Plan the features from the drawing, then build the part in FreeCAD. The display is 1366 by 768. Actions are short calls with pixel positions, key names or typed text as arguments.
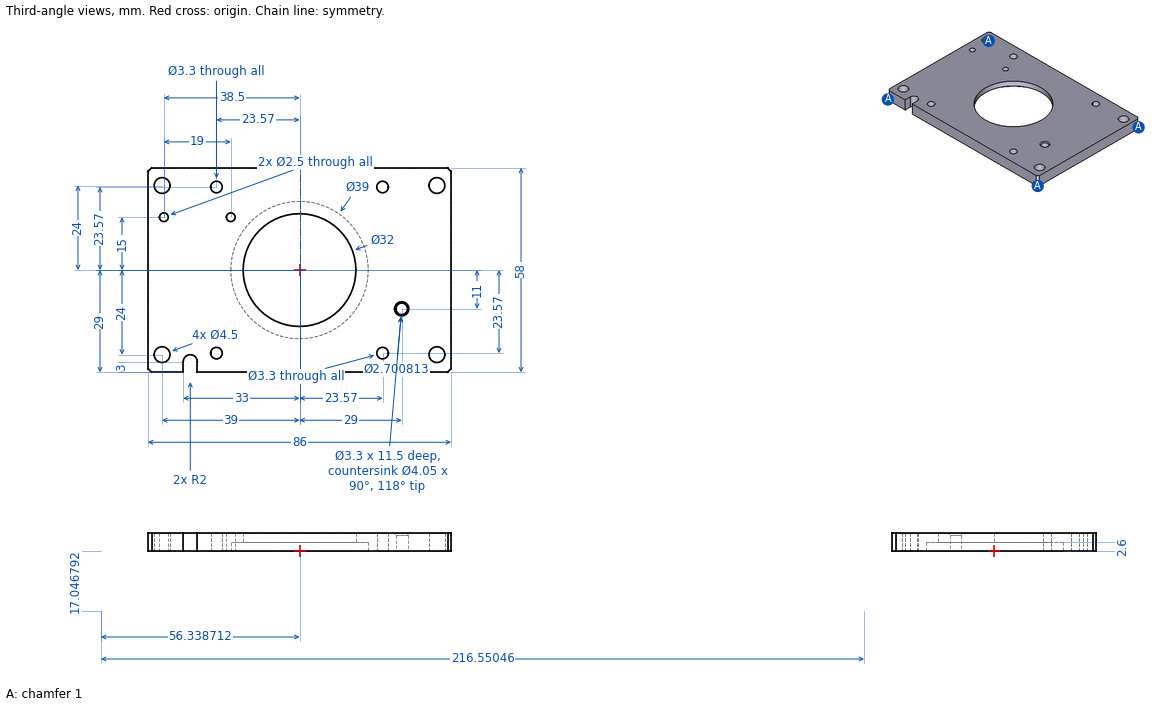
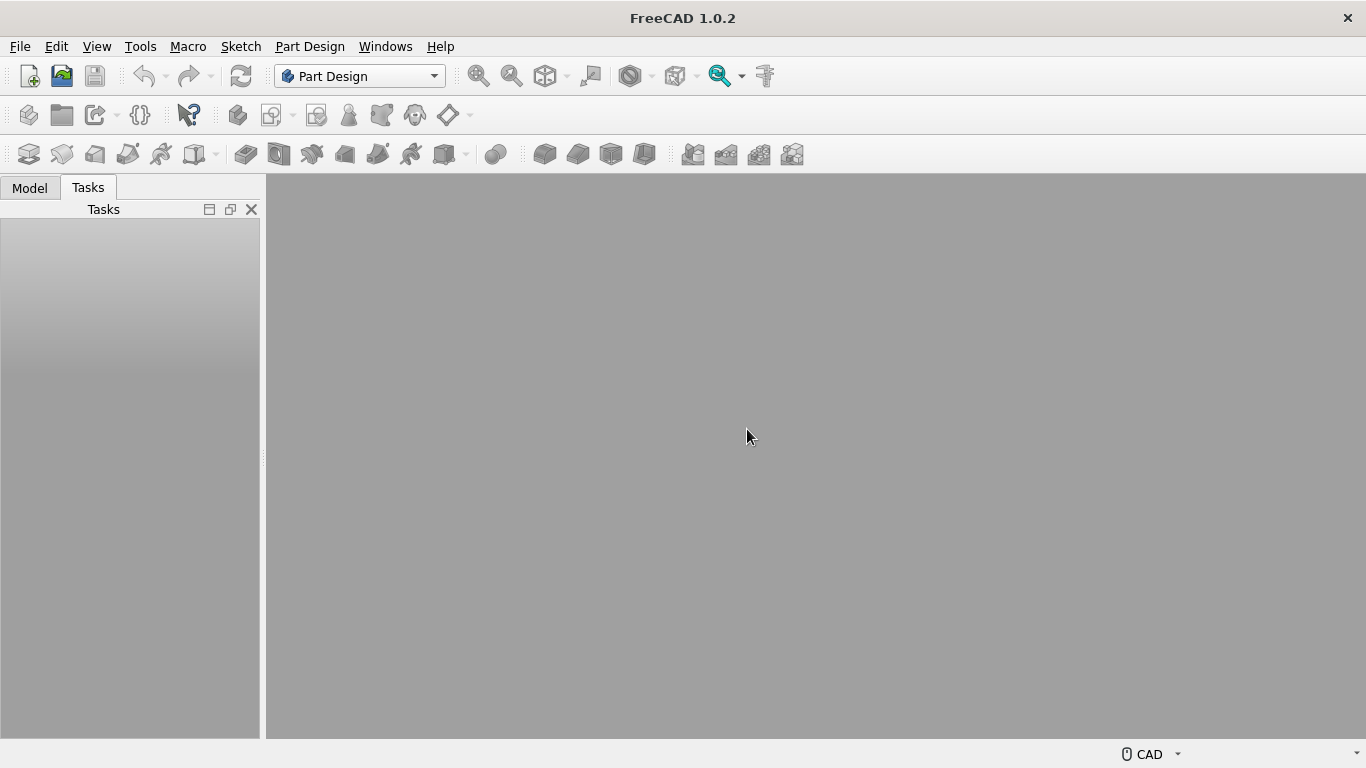
click(29, 76)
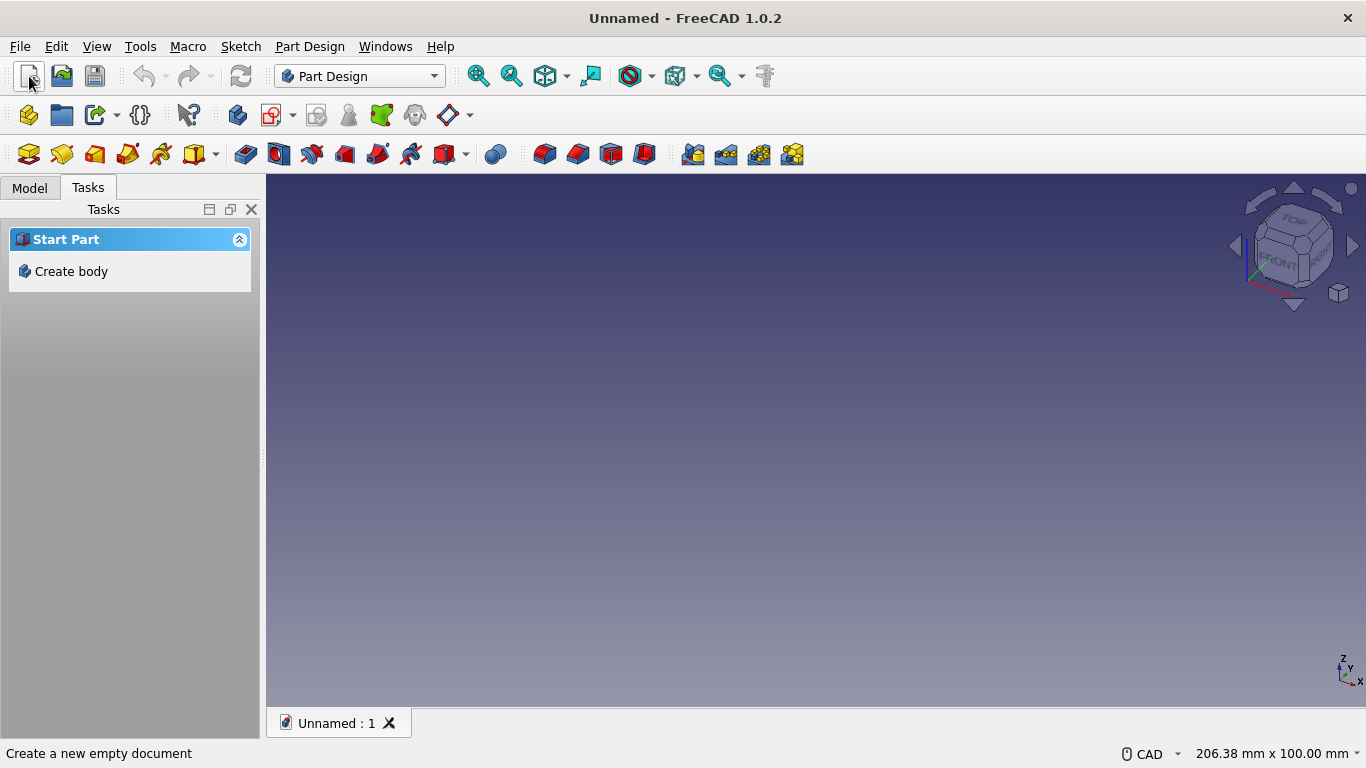
click(270, 116)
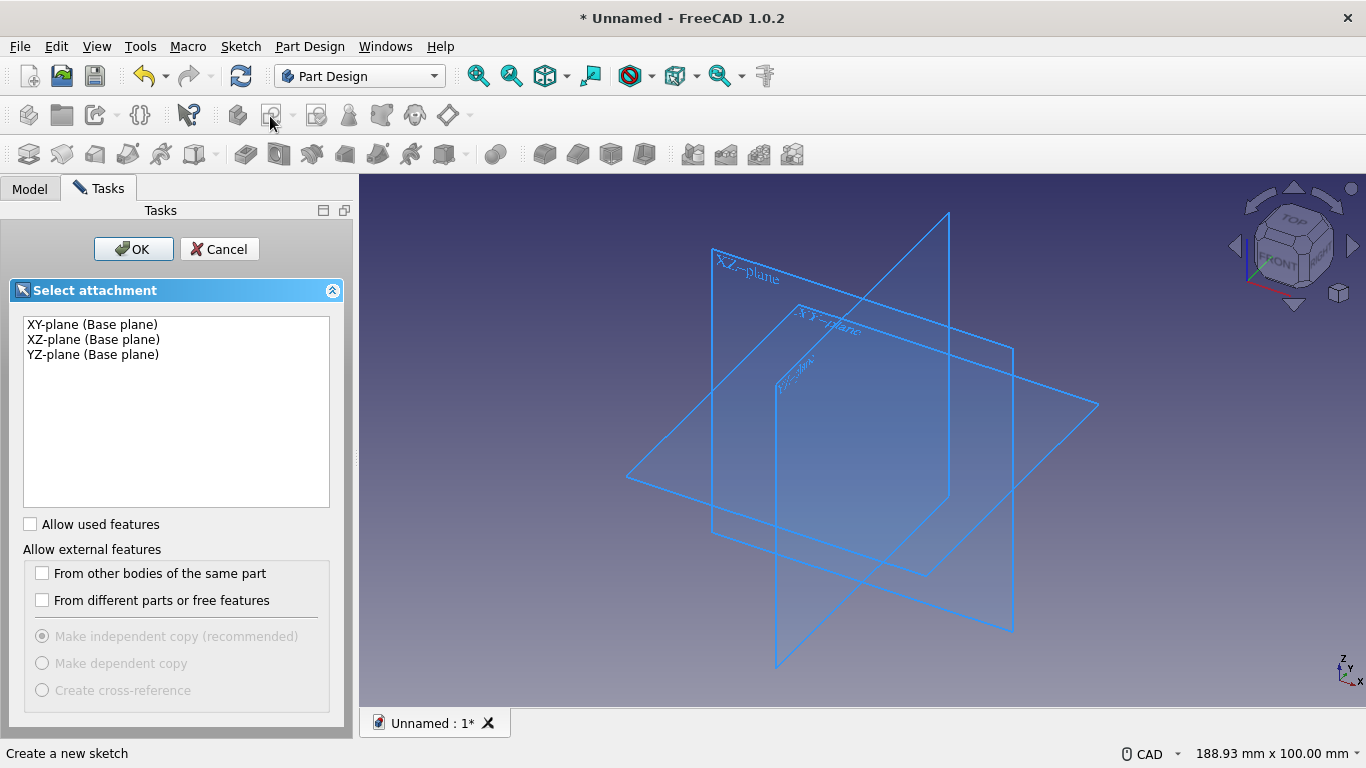
click(84, 324)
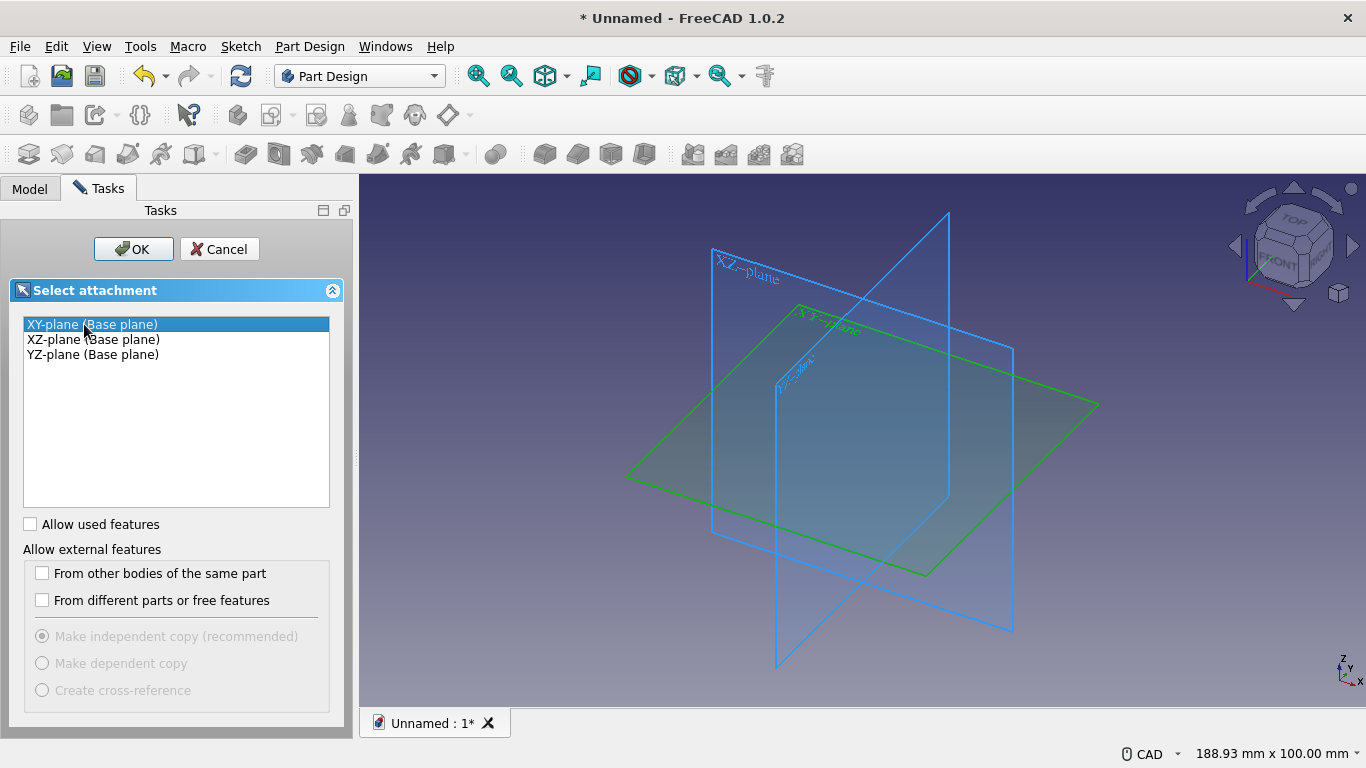
click(134, 249)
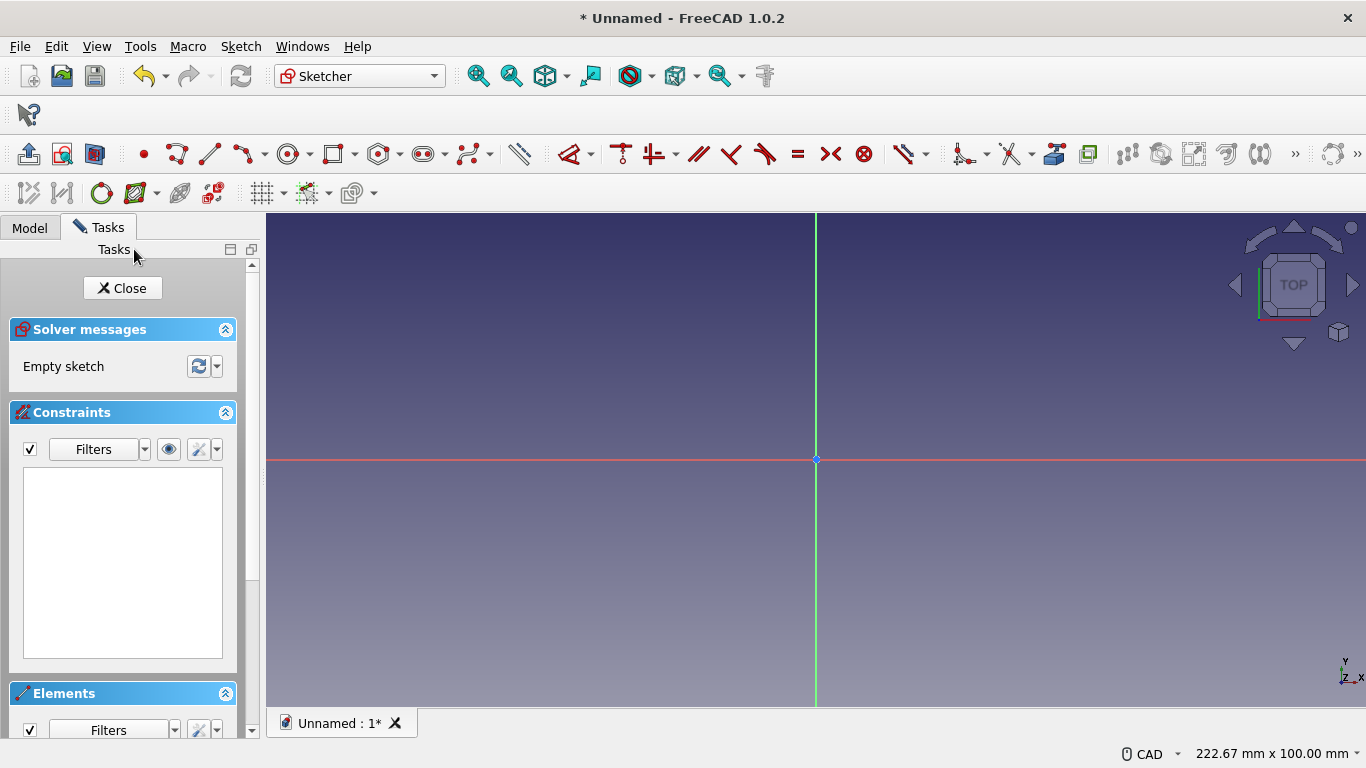
key(g)
key(v)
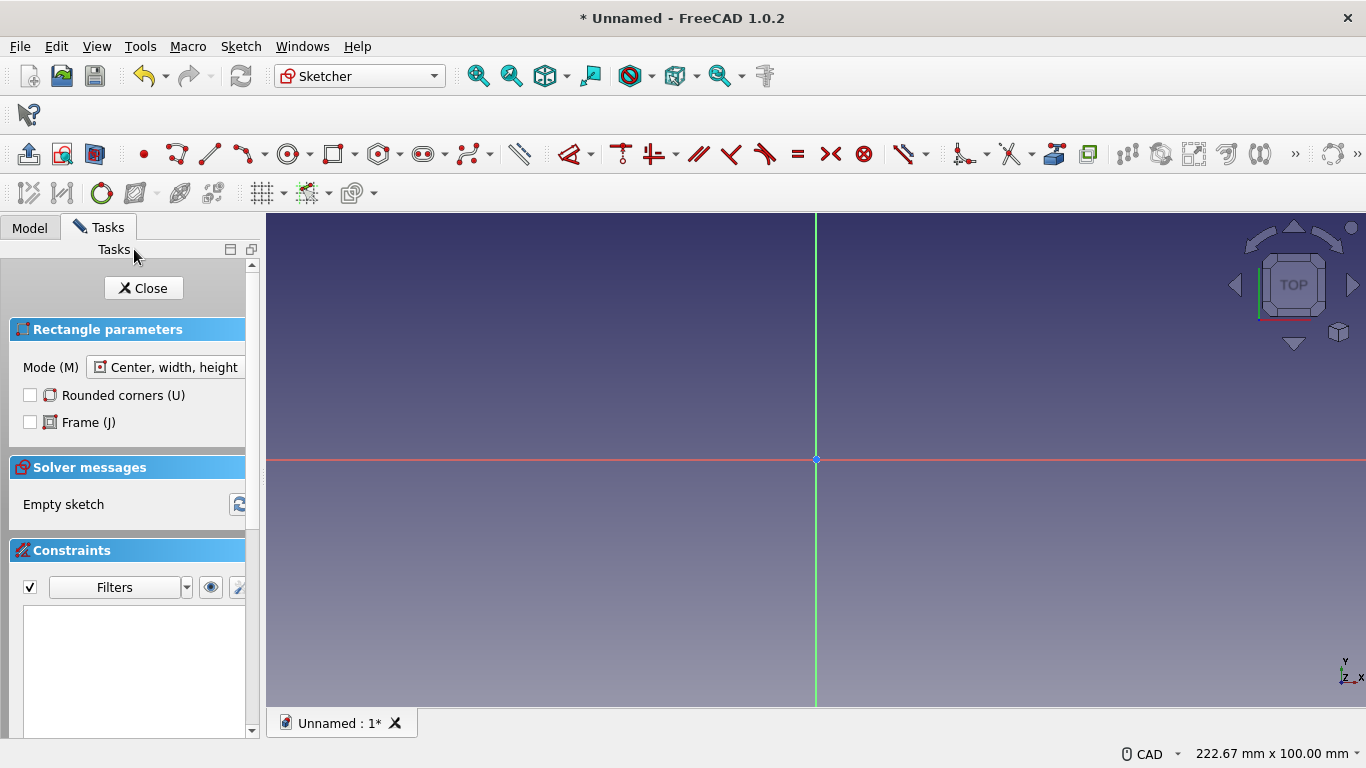
click(816, 460)
move(1028, 317)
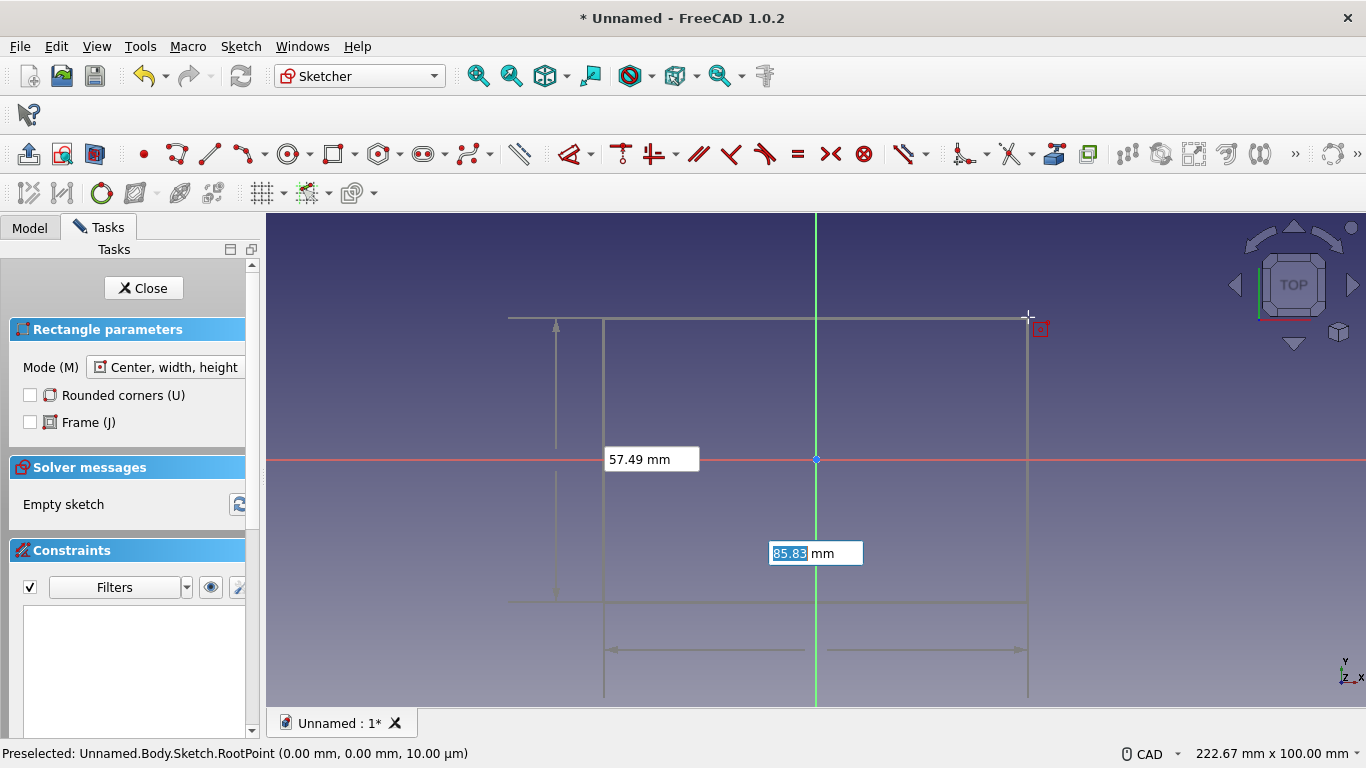
text(86)
key(Tab)
text(58)
key(Return)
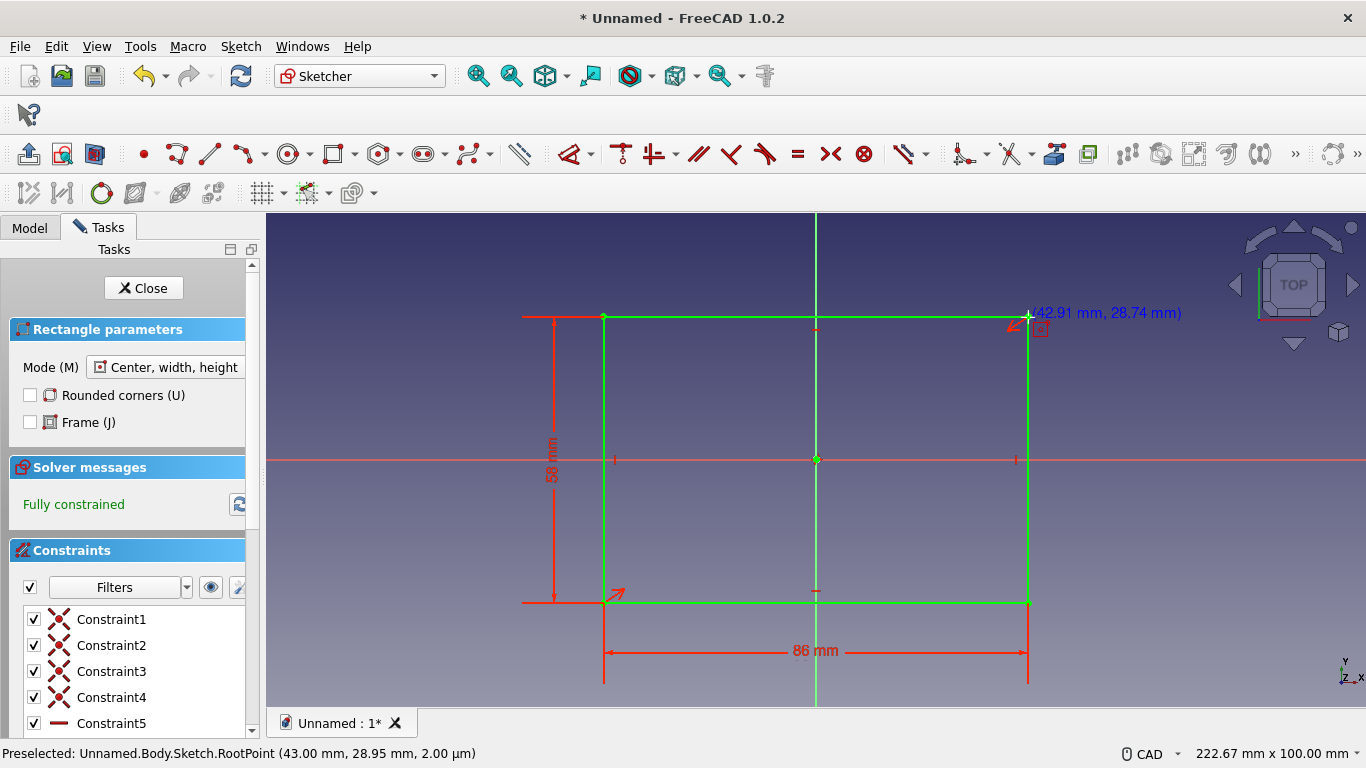
key(g)
key(c)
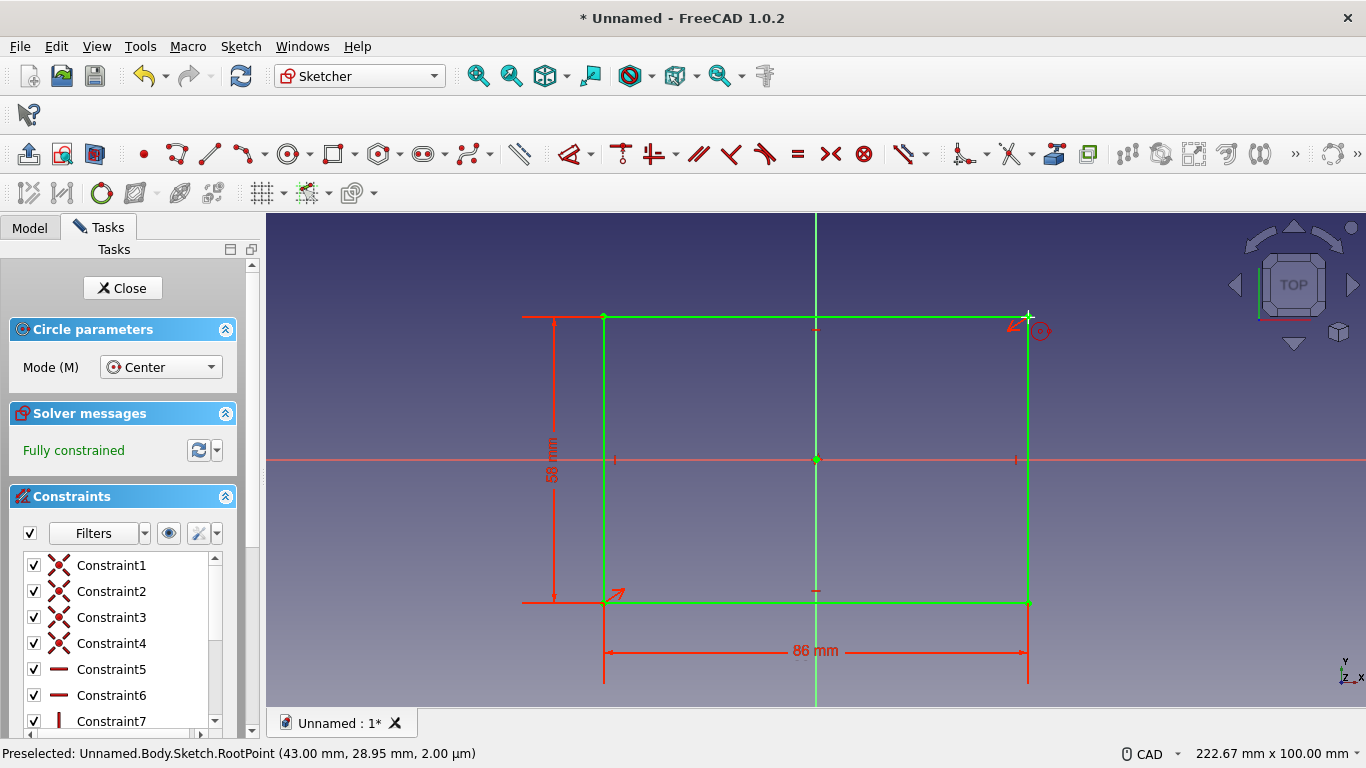
scroll(623, 579, up, 4)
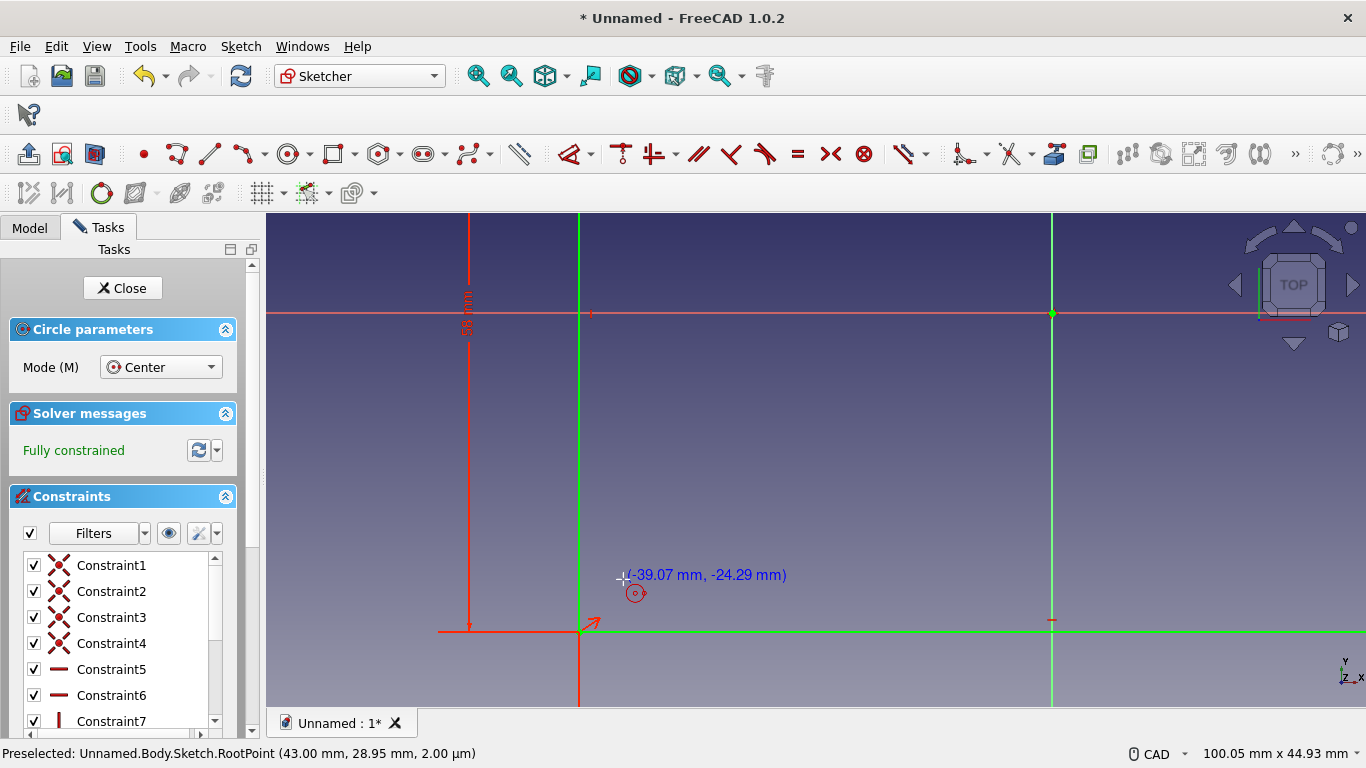
click(623, 577)
move(641, 560)